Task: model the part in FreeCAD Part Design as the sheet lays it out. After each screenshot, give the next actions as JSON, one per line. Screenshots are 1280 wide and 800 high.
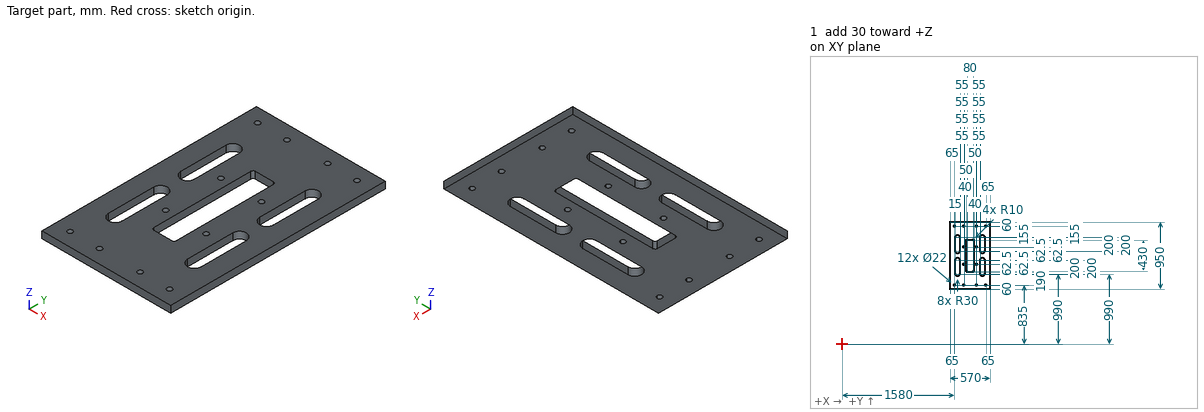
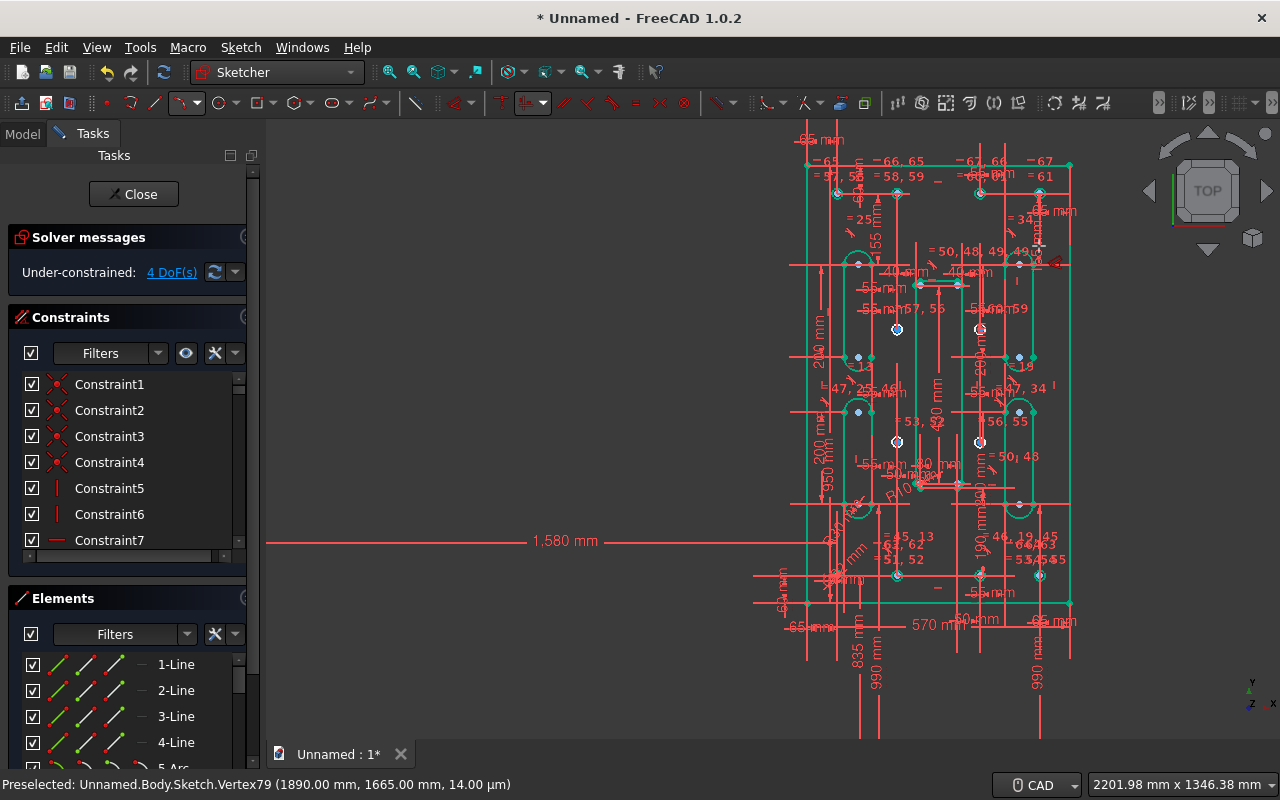
{"action": "scroll", "coordinate": [872, 412], "scroll_direction": "up", "scroll_amount": 2}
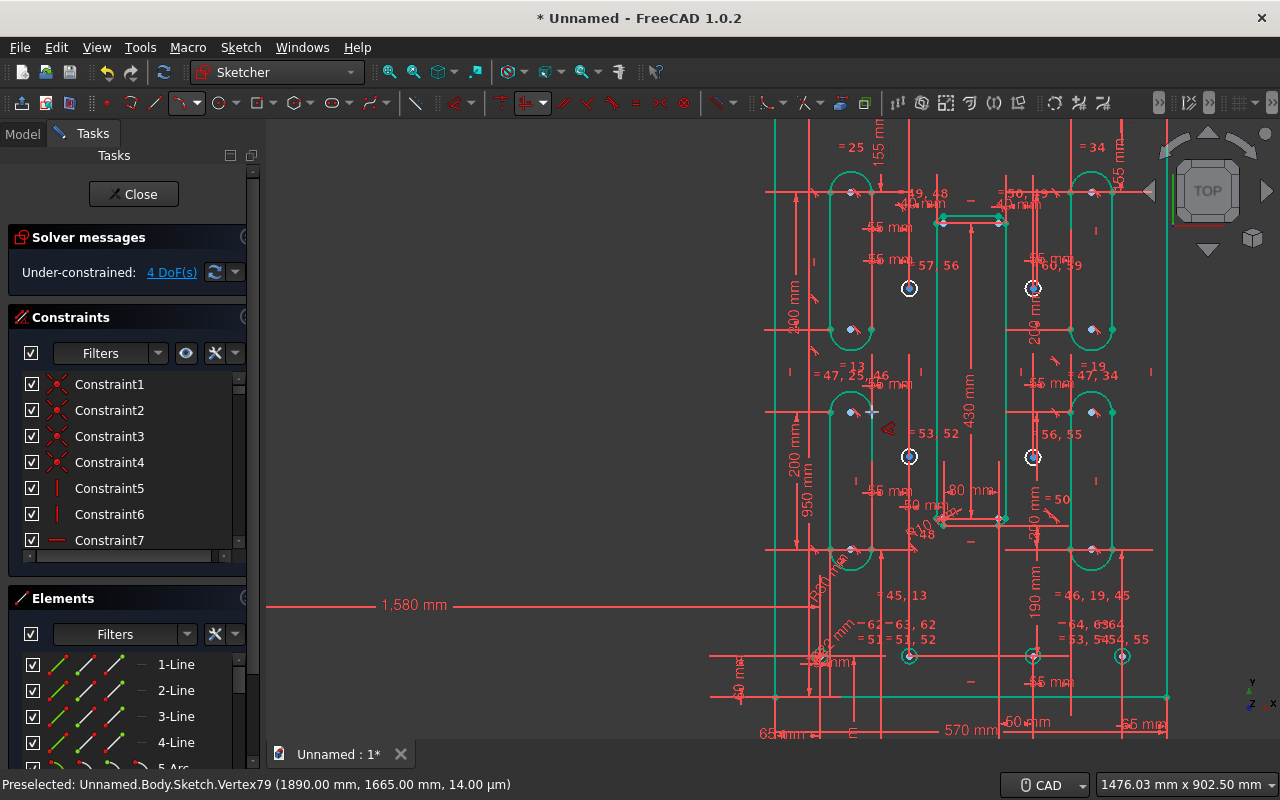
{"action": "left_click", "coordinate": [872, 412]}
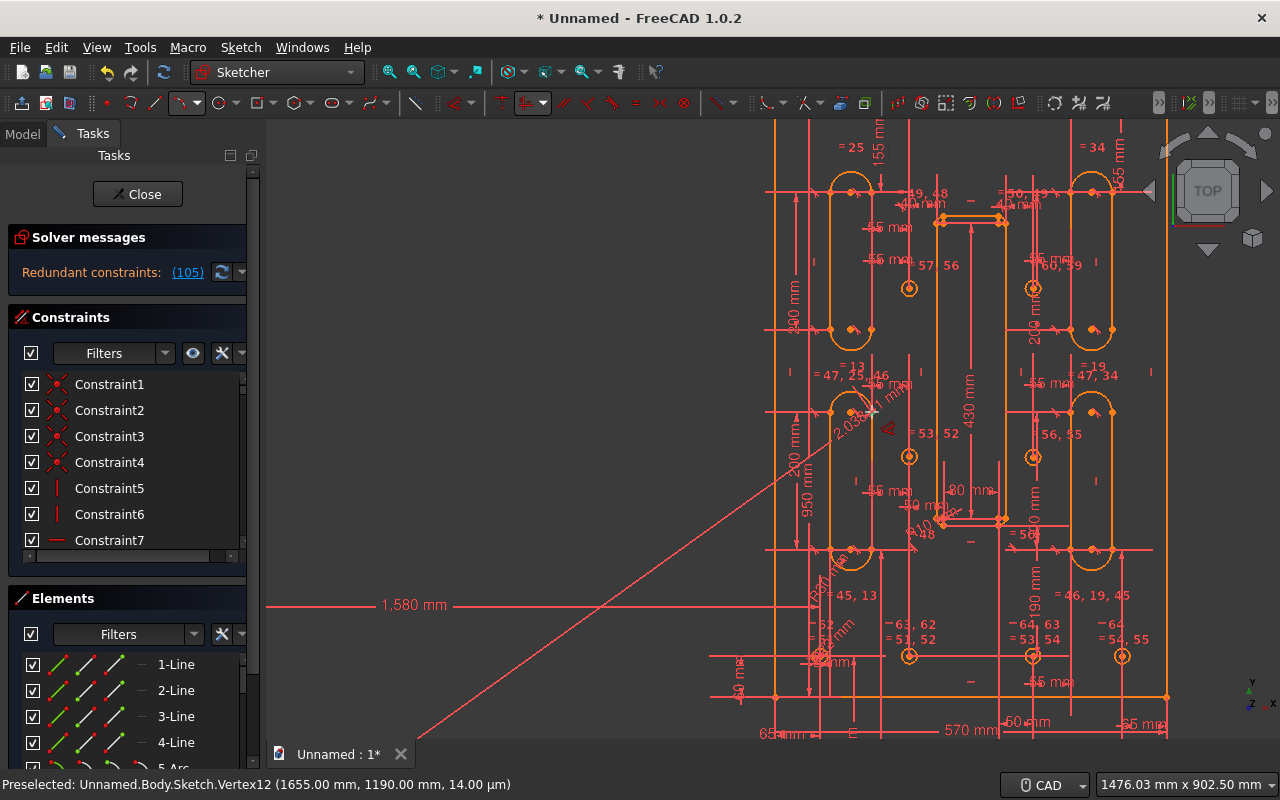
{"action": "left_click", "coordinate": [909, 457]}
{"action": "left_click", "coordinate": [967, 435]}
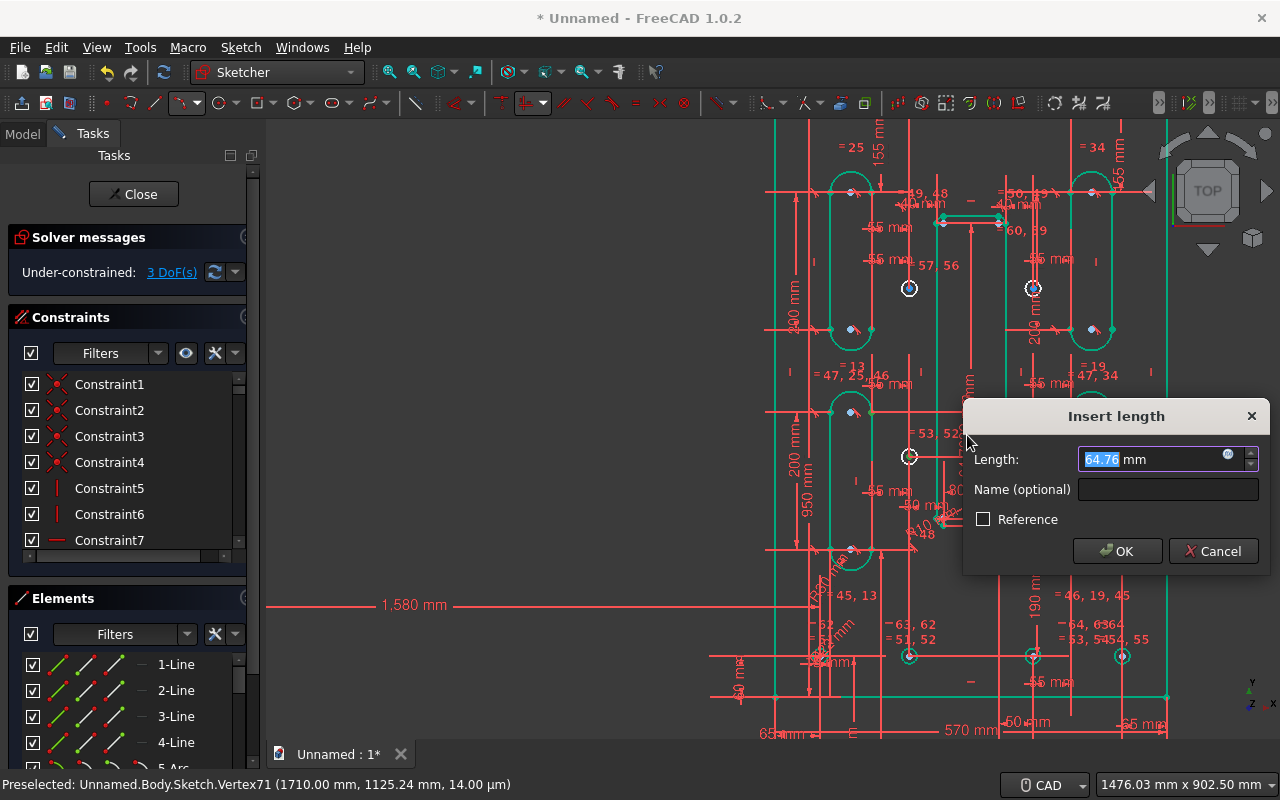
{"action": "type", "text": "62.5"}
{"action": "key", "text": "Return"}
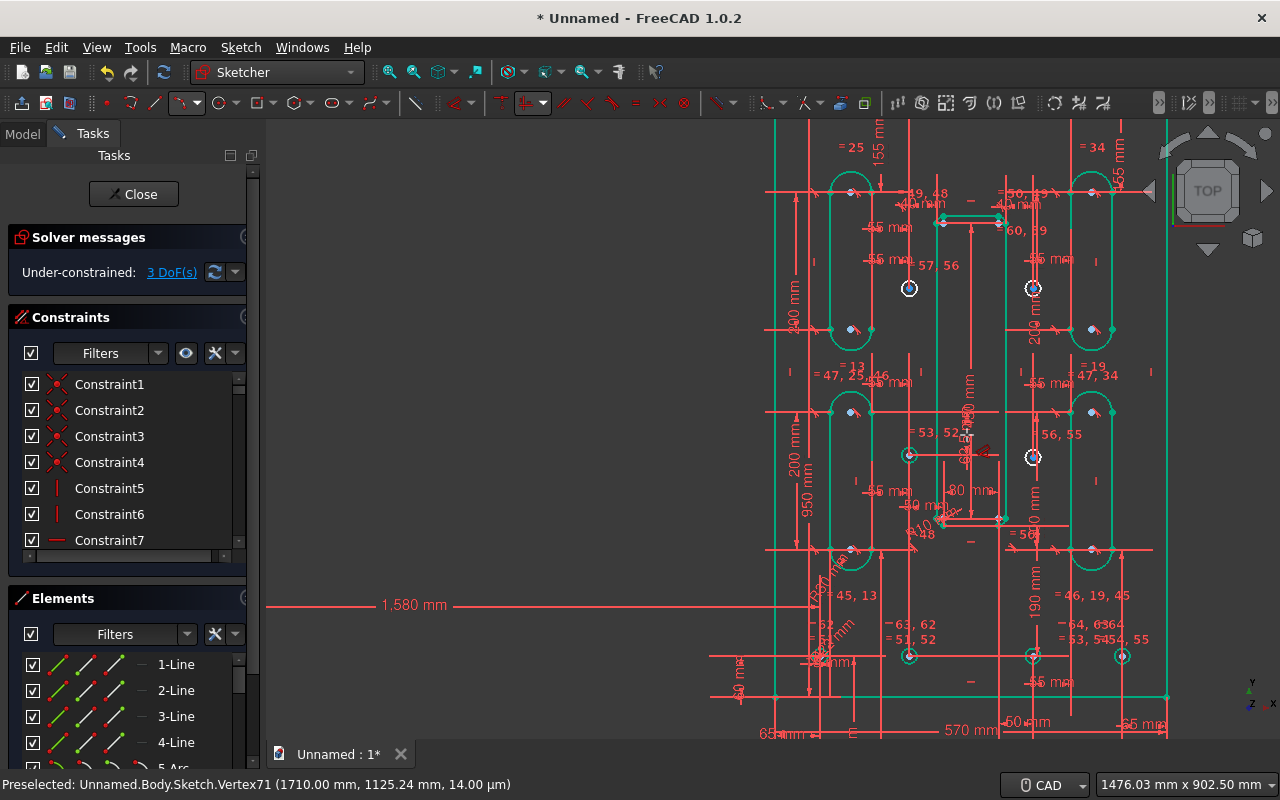
{"action": "left_click", "coordinate": [1071, 412]}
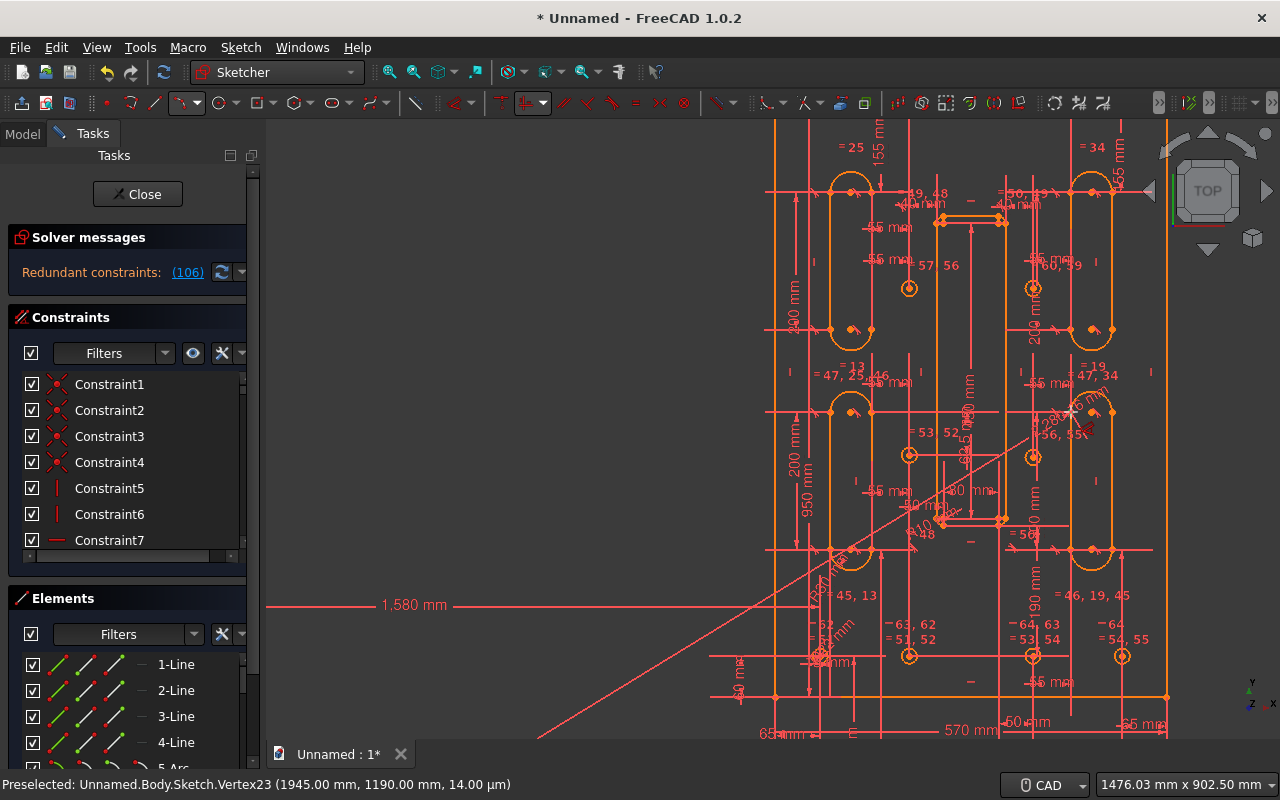
{"action": "left_click", "coordinate": [1033, 457]}
{"action": "left_click", "coordinate": [853, 424]}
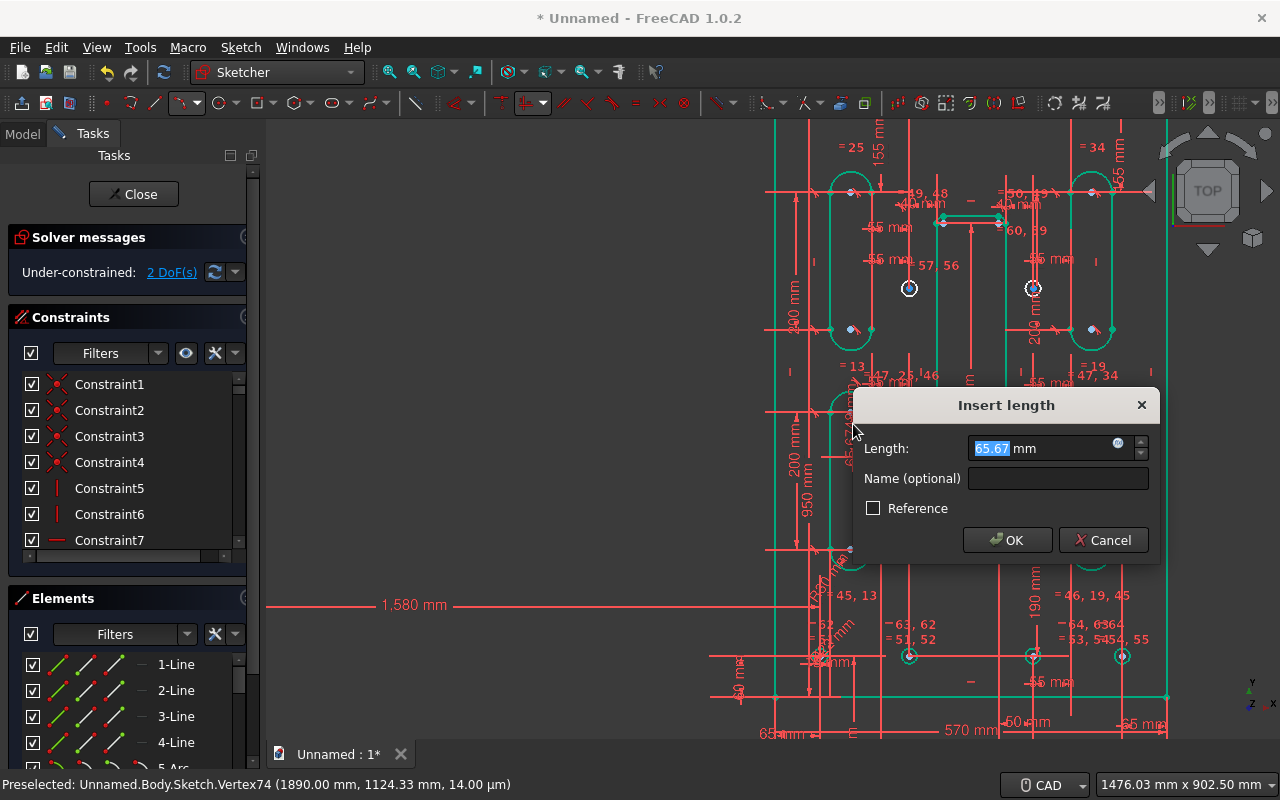
{"action": "type", "text": "62.5"}
{"action": "key", "text": "Return"}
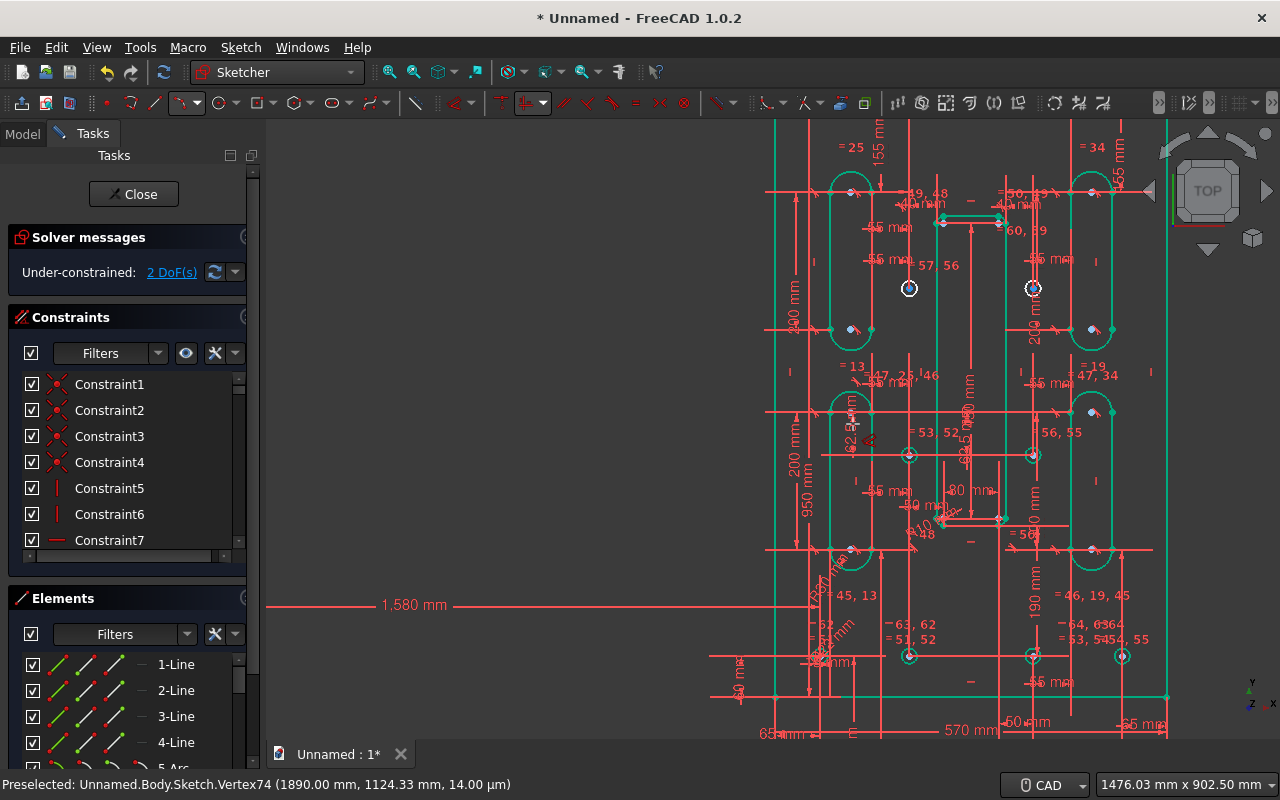
{"action": "left_click", "coordinate": [872, 330]}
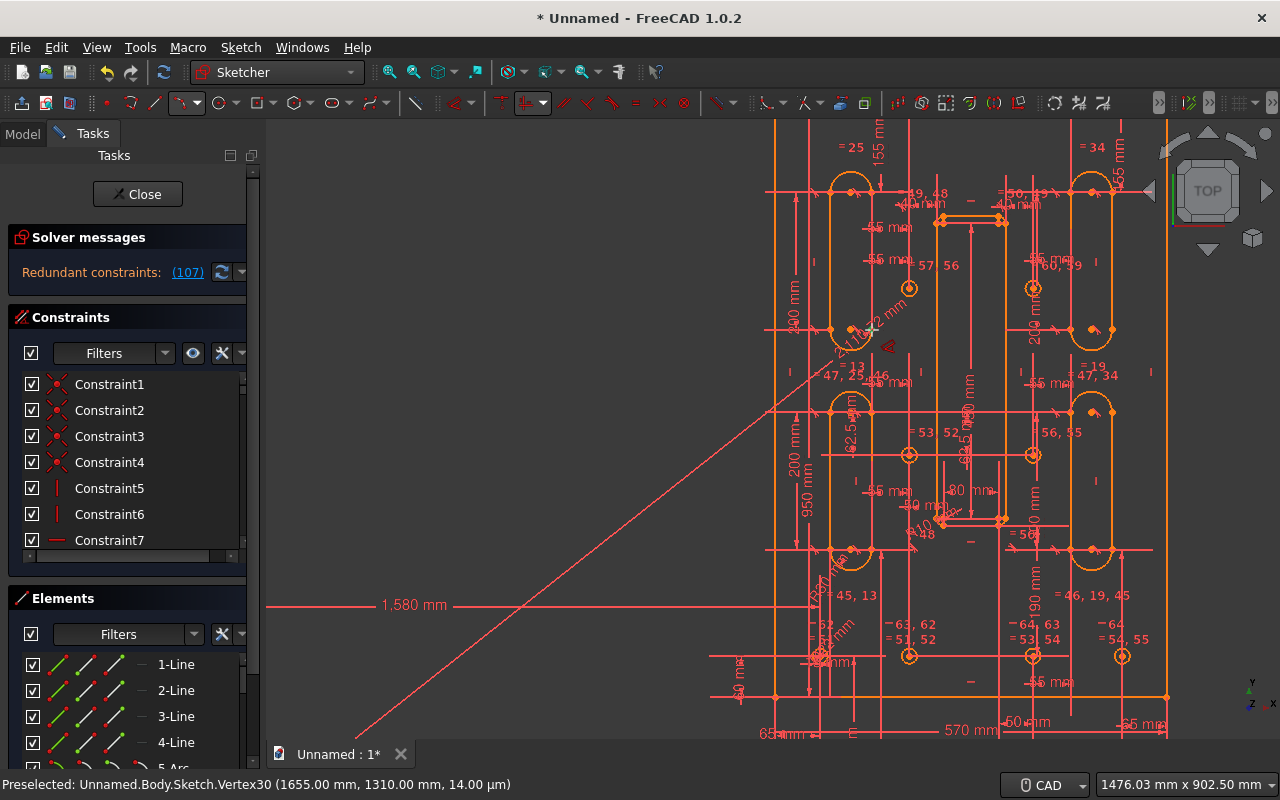
{"action": "left_click", "coordinate": [909, 289]}
{"action": "left_click", "coordinate": [967, 295]}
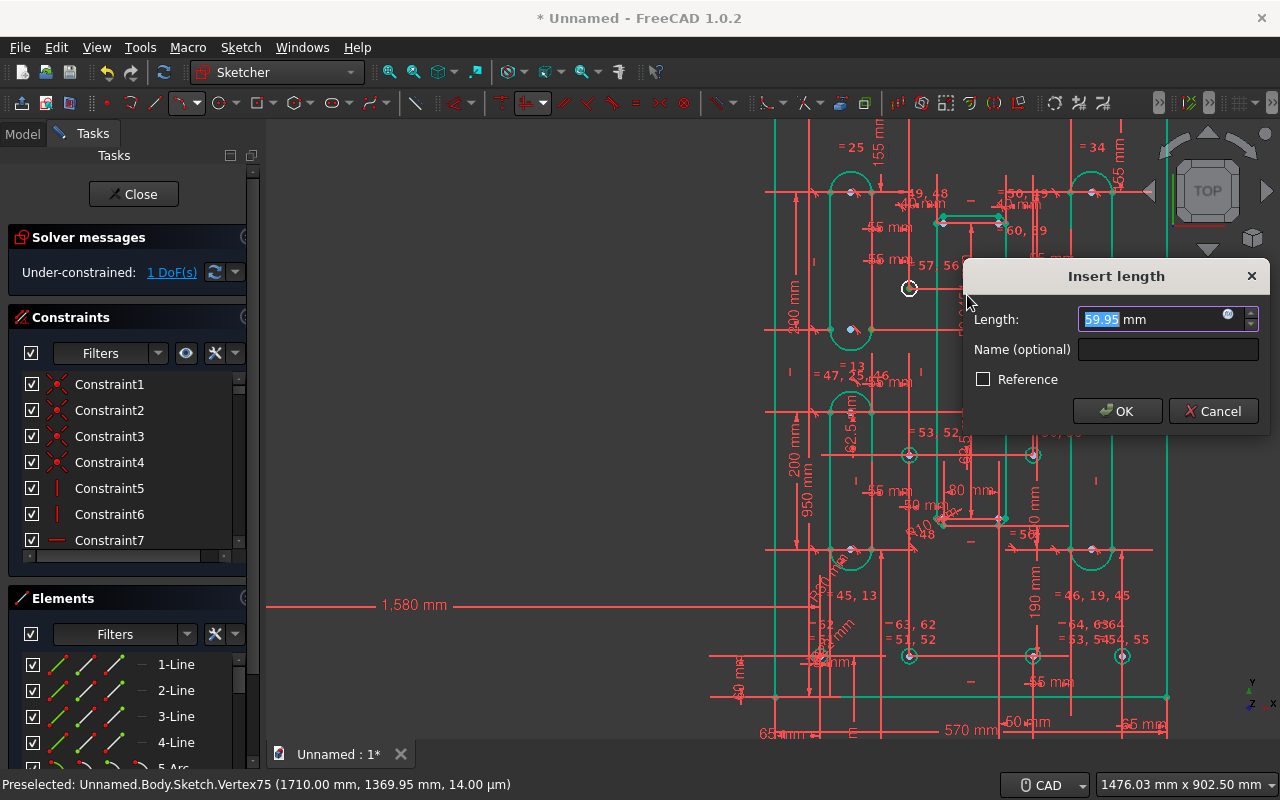
{"action": "type", "text": "62.5"}
{"action": "key", "text": "Return"}